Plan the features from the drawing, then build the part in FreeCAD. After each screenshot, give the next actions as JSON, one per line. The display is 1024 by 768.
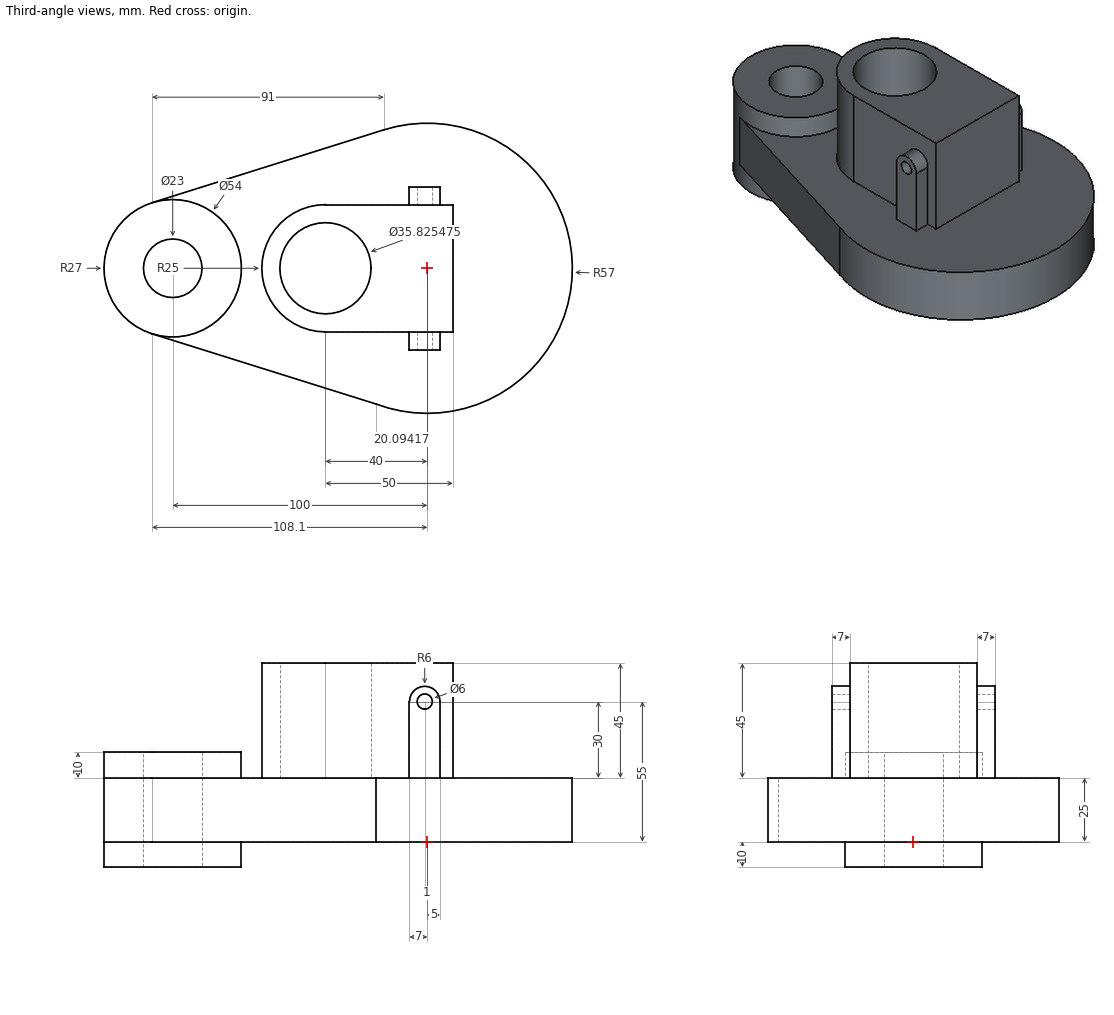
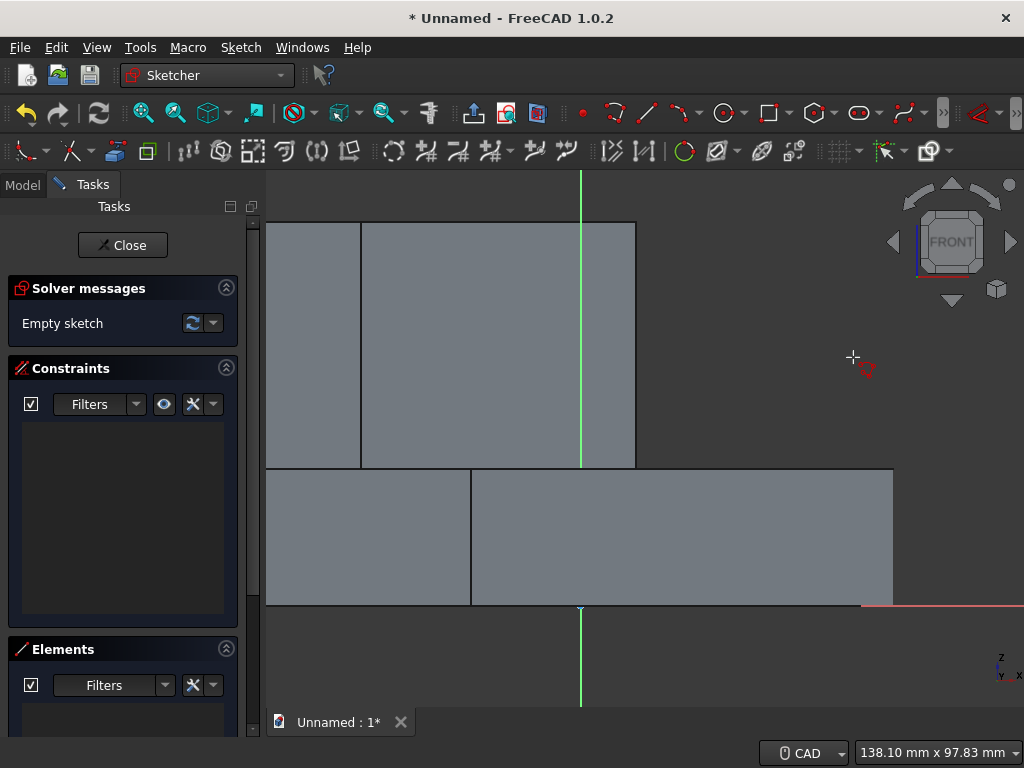
{"action": "left_click", "coordinate": [542, 304]}
{"action": "left_click", "coordinate": [542, 469]}
{"action": "left_click", "coordinate": [608, 469]}
{"action": "left_click", "coordinate": [608, 304]}
{"action": "right_click", "coordinate": [608, 304]}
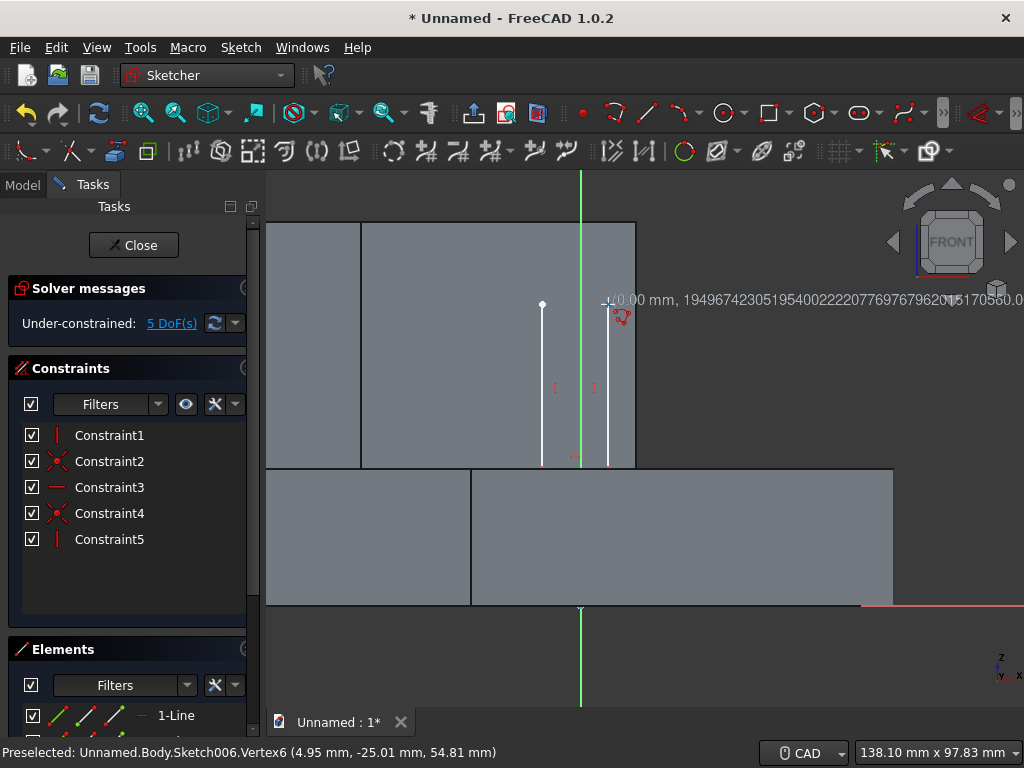
{"action": "left_click", "coordinate": [680, 114]}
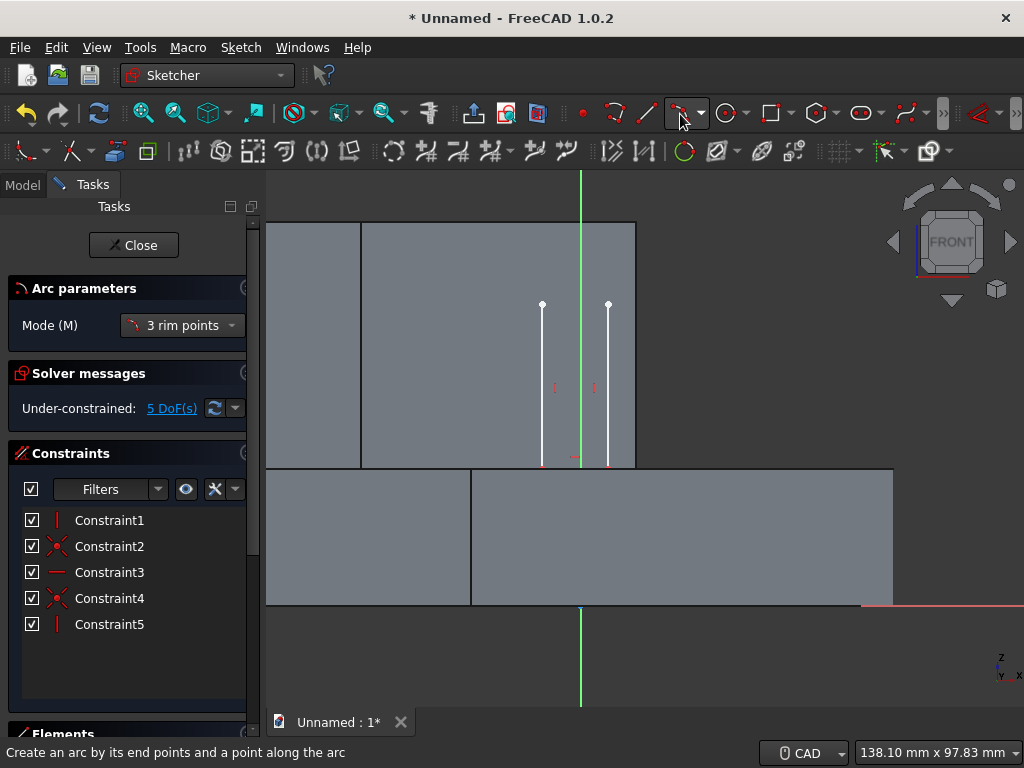
{"action": "left_click", "coordinate": [608, 305]}
{"action": "left_click", "coordinate": [542, 305]}
{"action": "left_click", "coordinate": [565, 273]}
{"action": "key", "text": "Escape"}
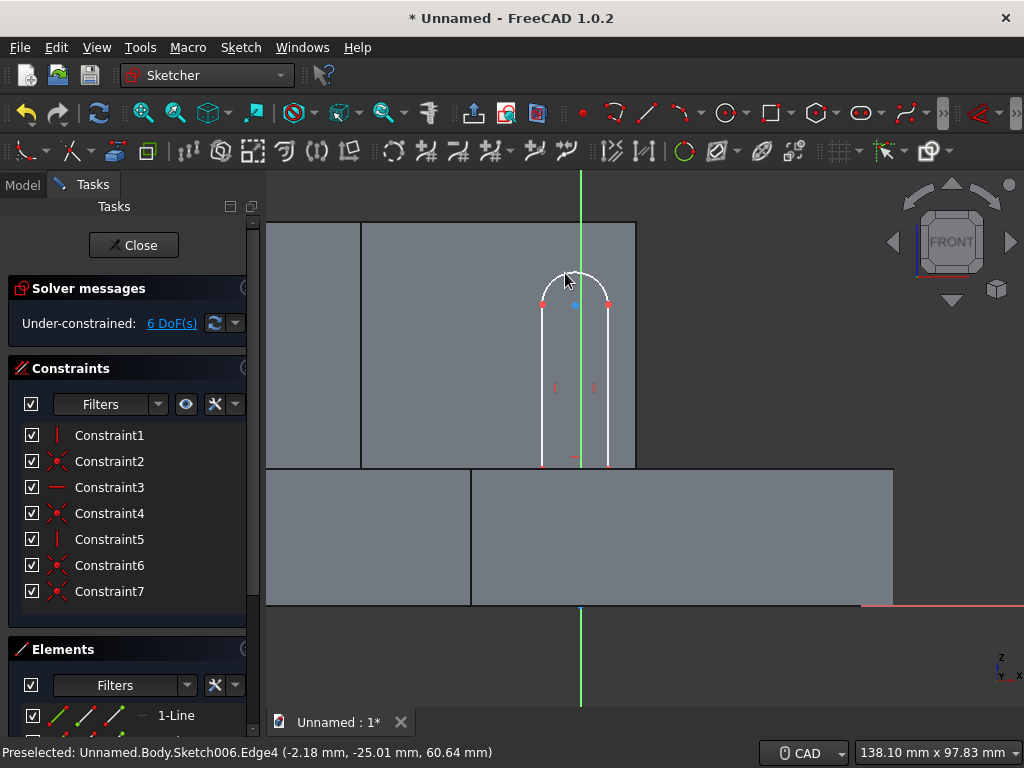
{"action": "left_click", "coordinate": [542, 355]}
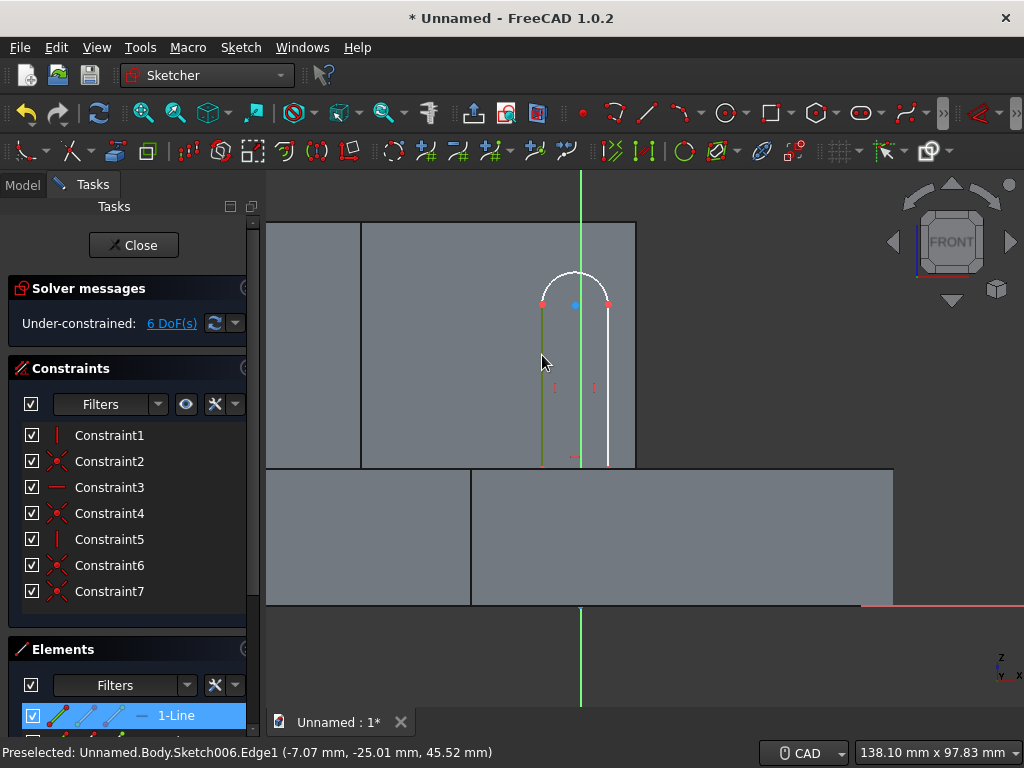
{"action": "left_click", "coordinate": [594, 279]}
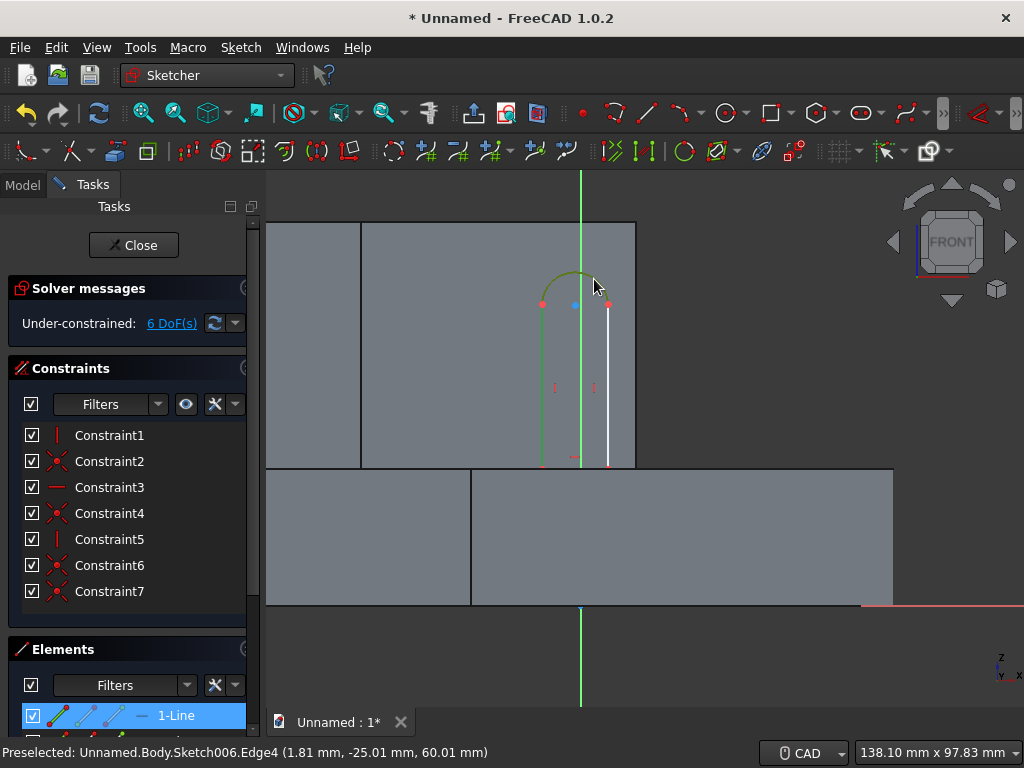
{"action": "key", "text": "t"}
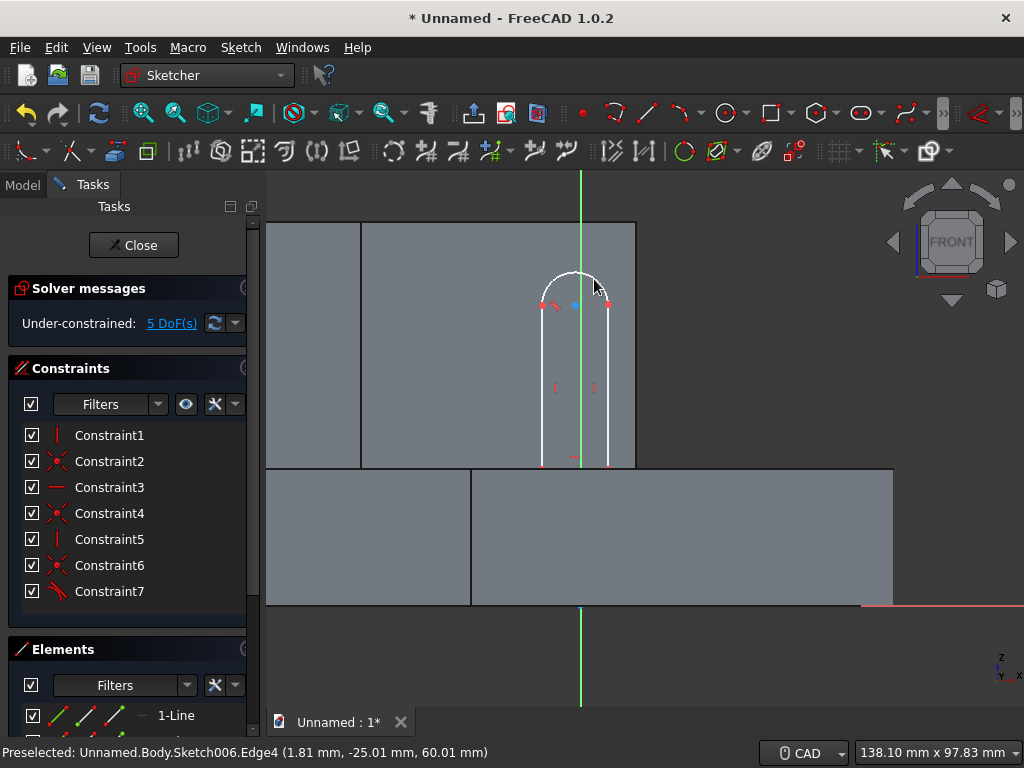
{"action": "left_click", "coordinate": [608, 421]}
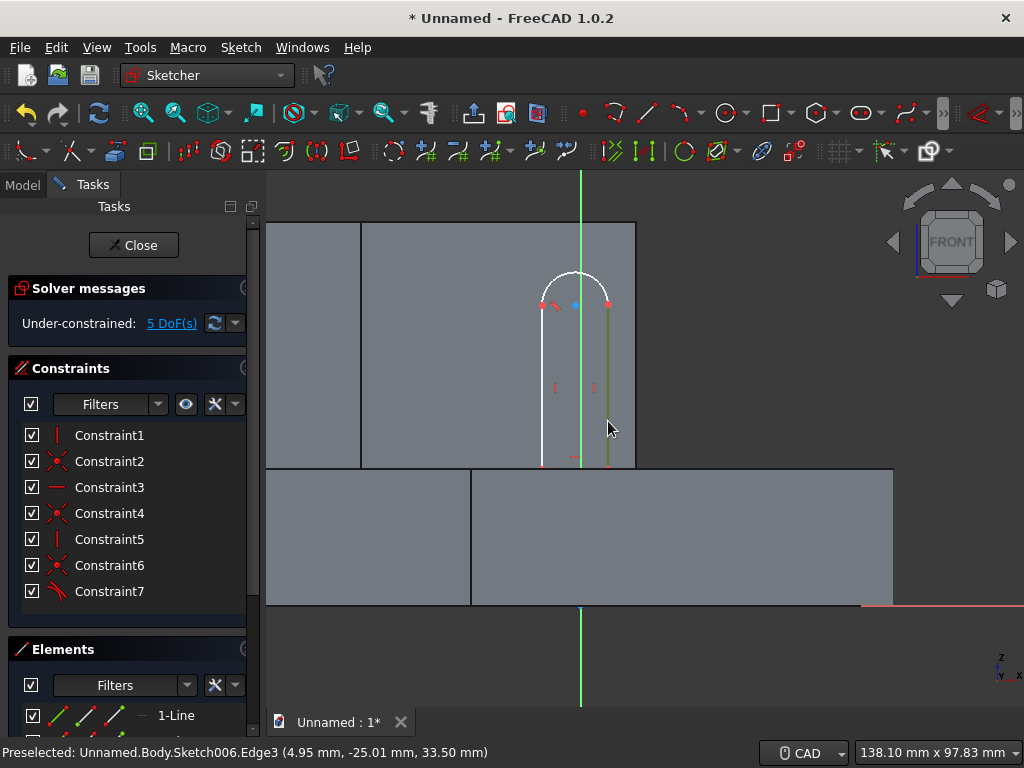
{"action": "left_click", "coordinate": [594, 279]}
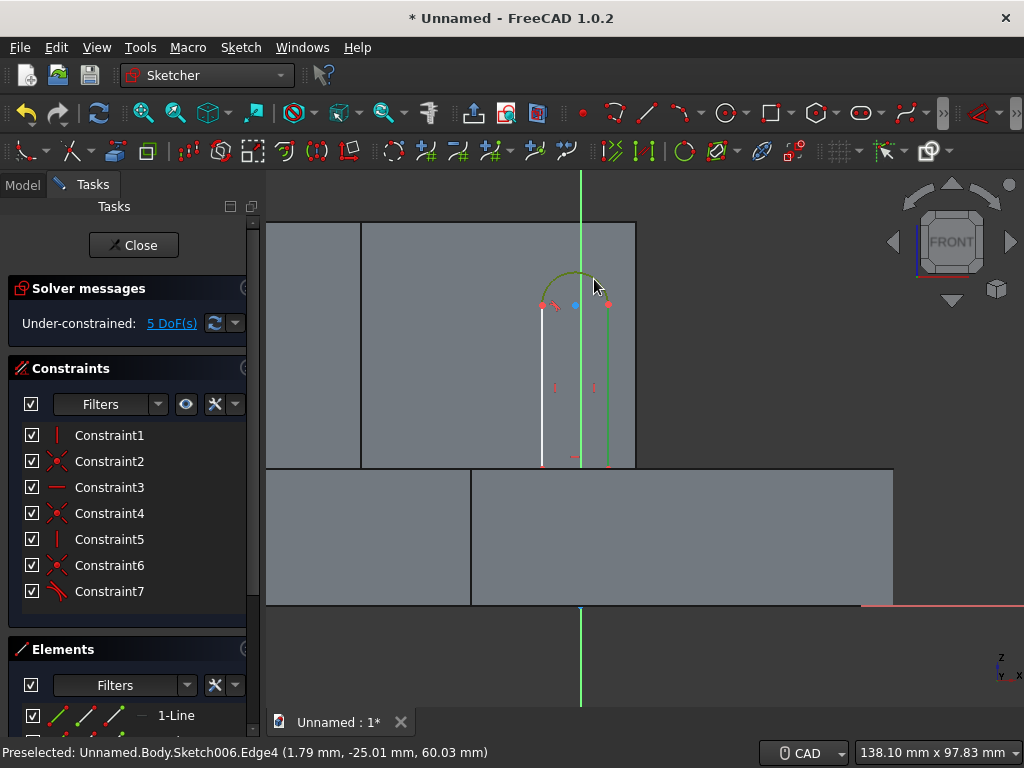
{"action": "key", "text": "t"}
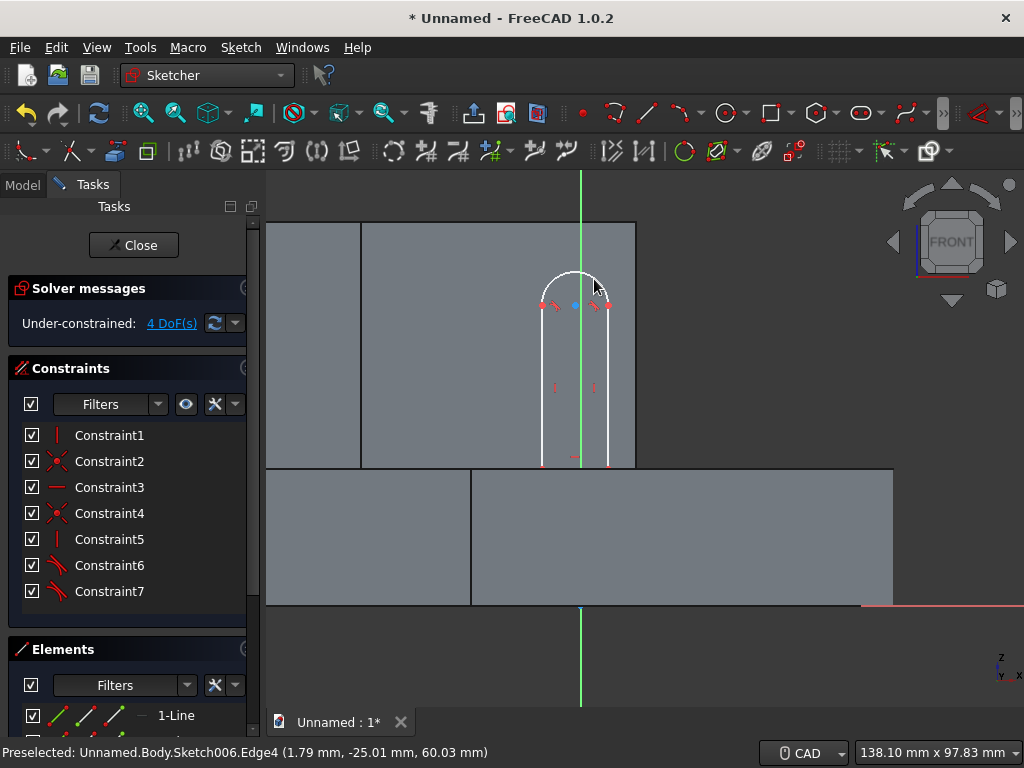
{"action": "left_click", "coordinate": [978, 114]}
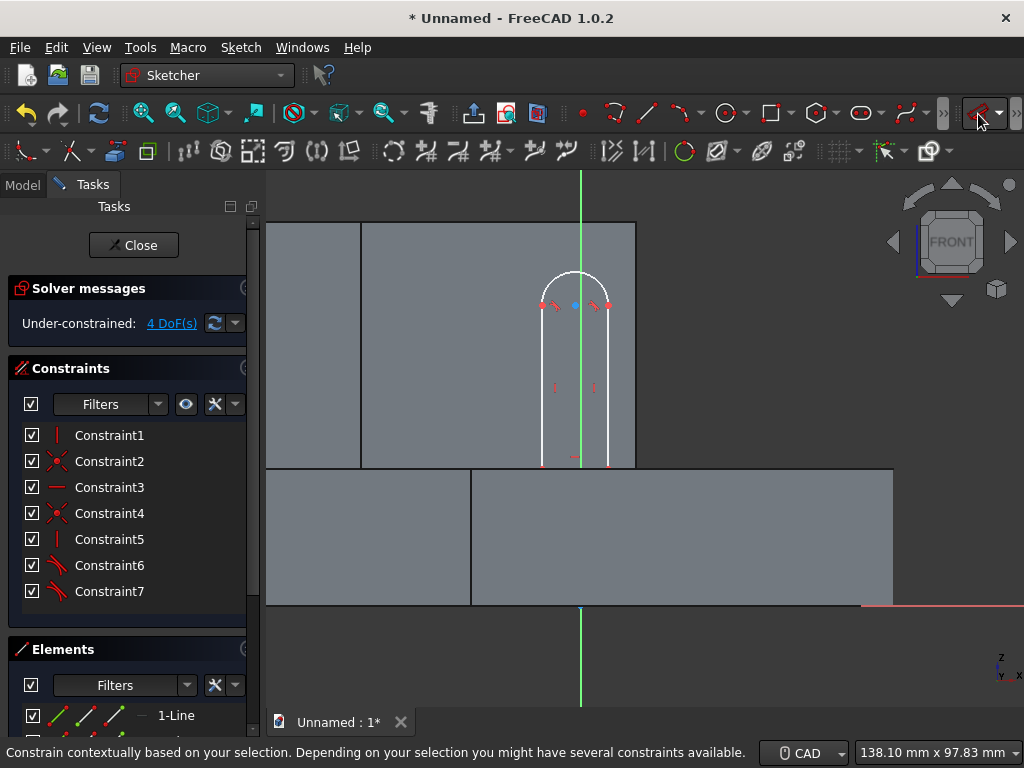
{"action": "left_click", "coordinate": [594, 278]}
{"action": "left_click", "coordinate": [612, 252]}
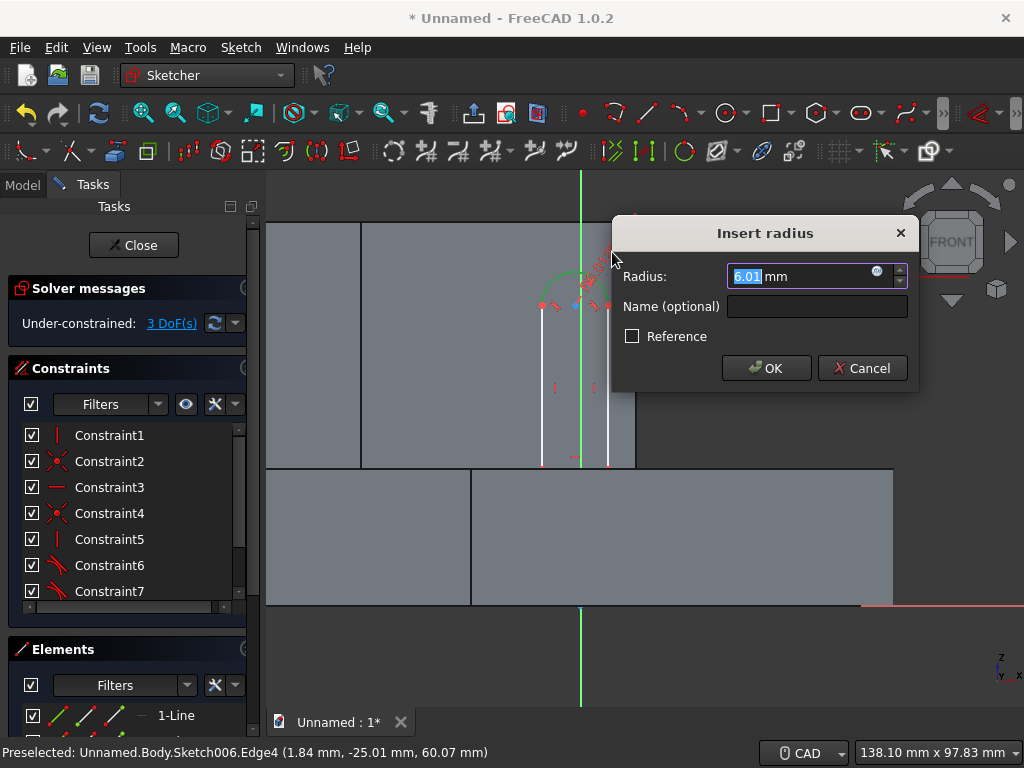
{"action": "type", "text": "6"}
{"action": "key", "text": "Return"}